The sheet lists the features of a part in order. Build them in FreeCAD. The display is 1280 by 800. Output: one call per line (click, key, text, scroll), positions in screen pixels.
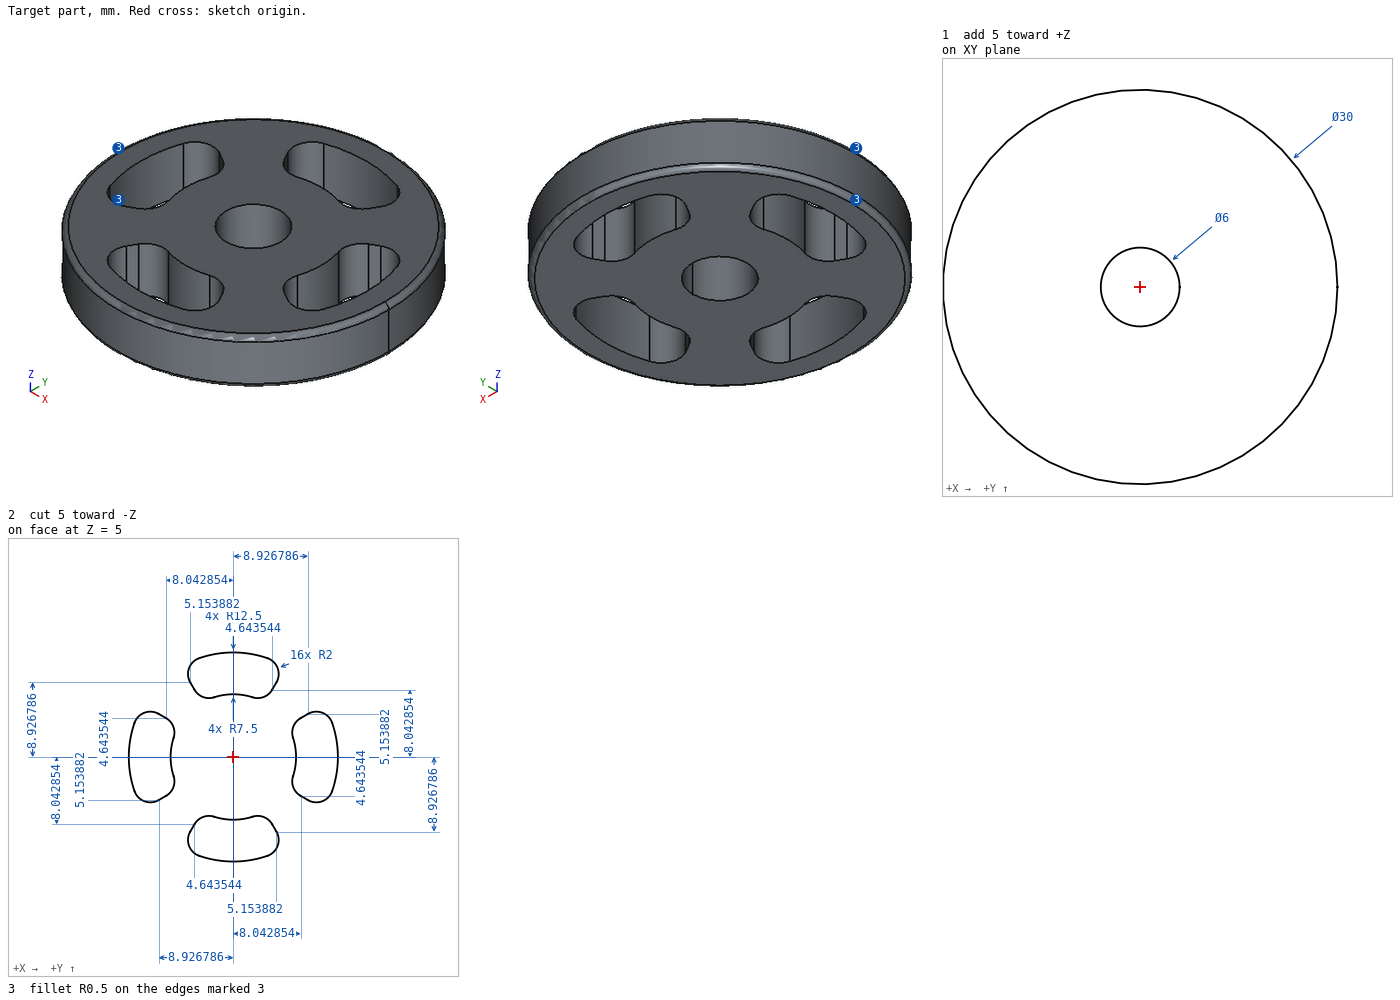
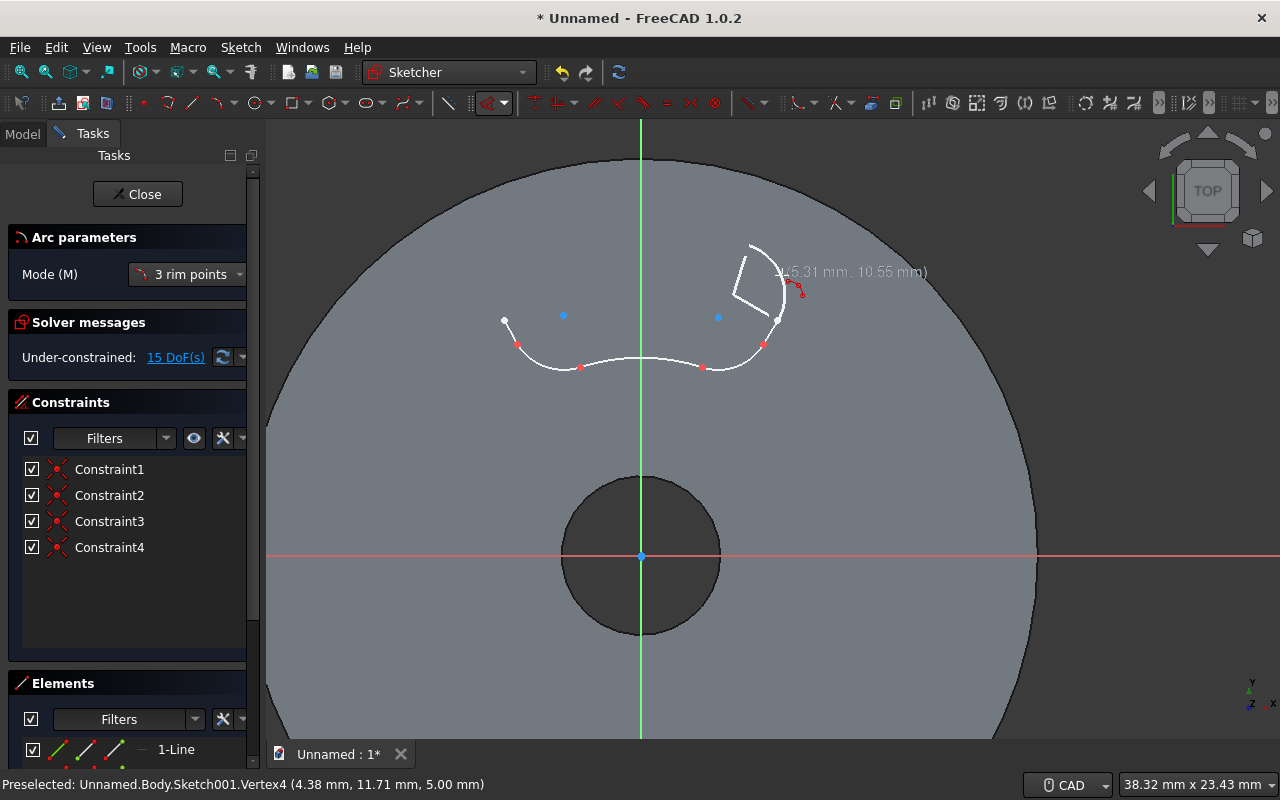
click(781, 274)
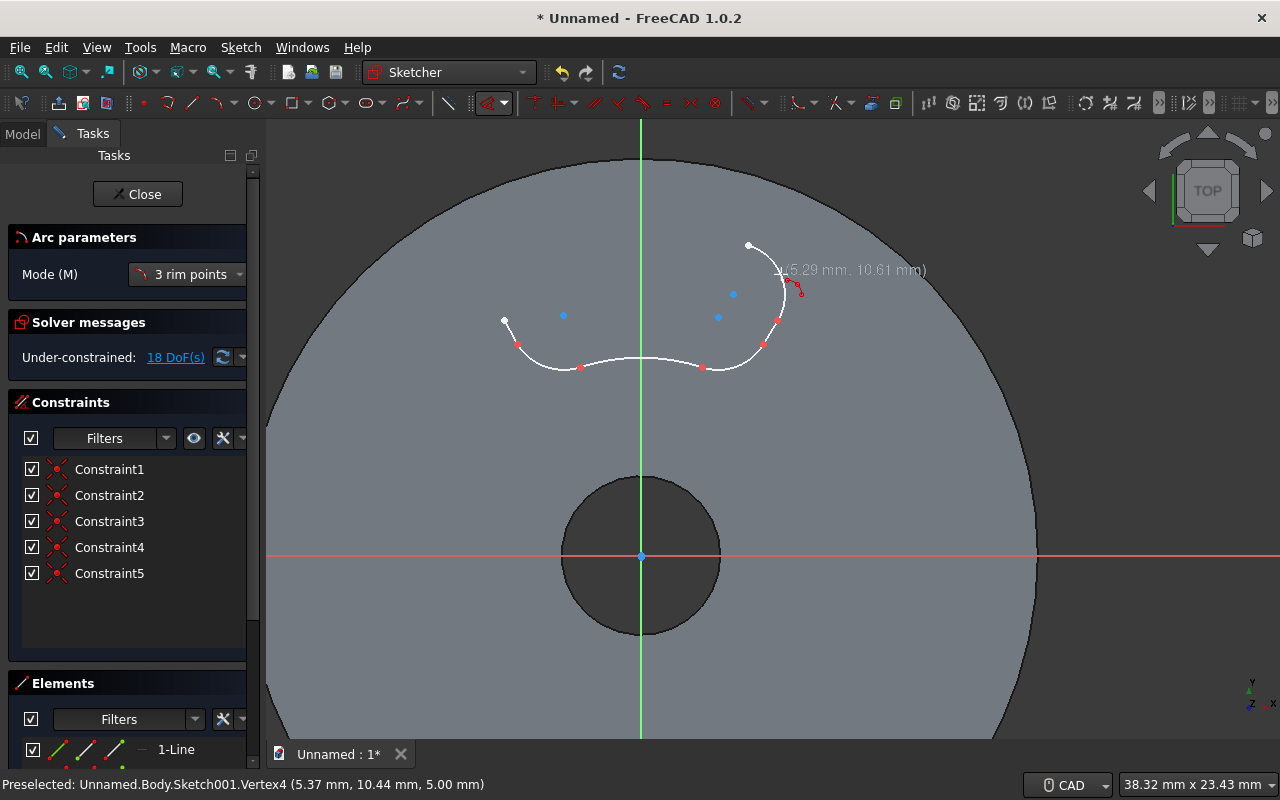
click(749, 246)
click(533, 243)
click(663, 226)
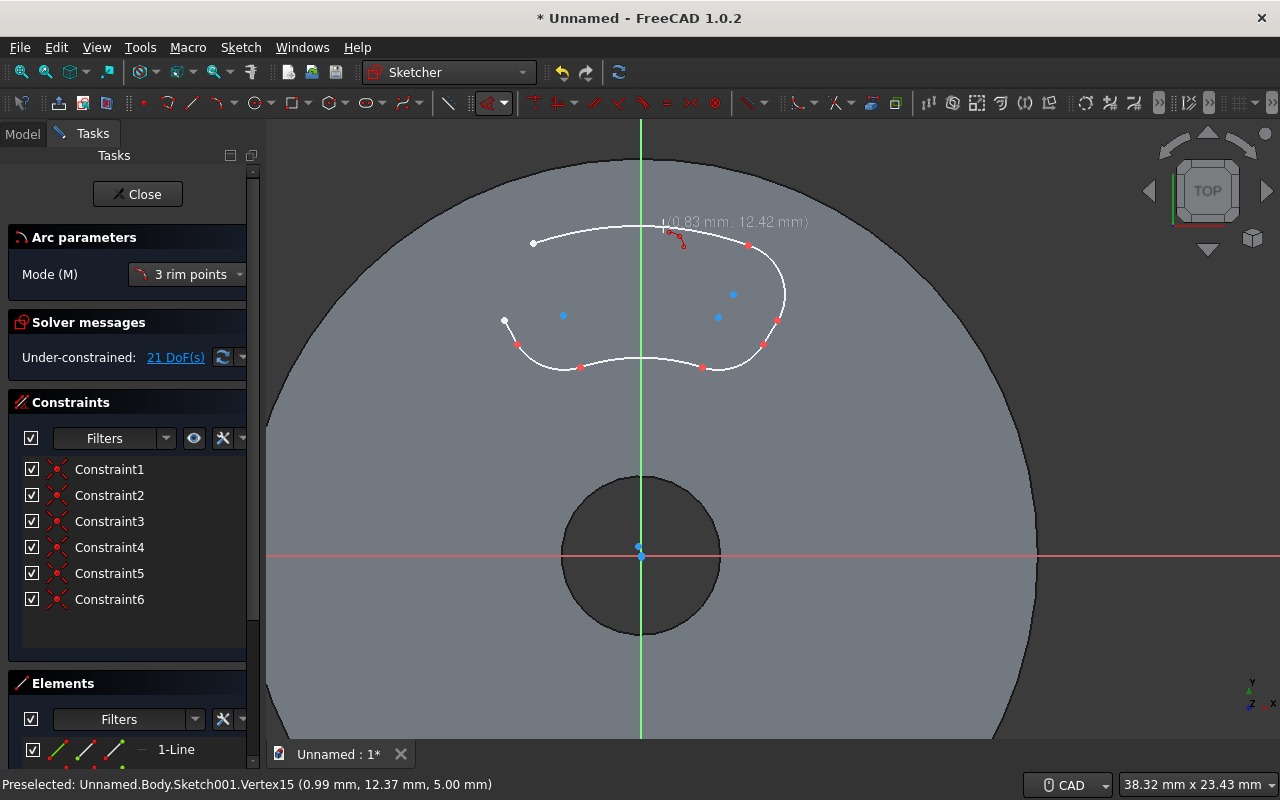
click(533, 244)
click(505, 321)
click(501, 274)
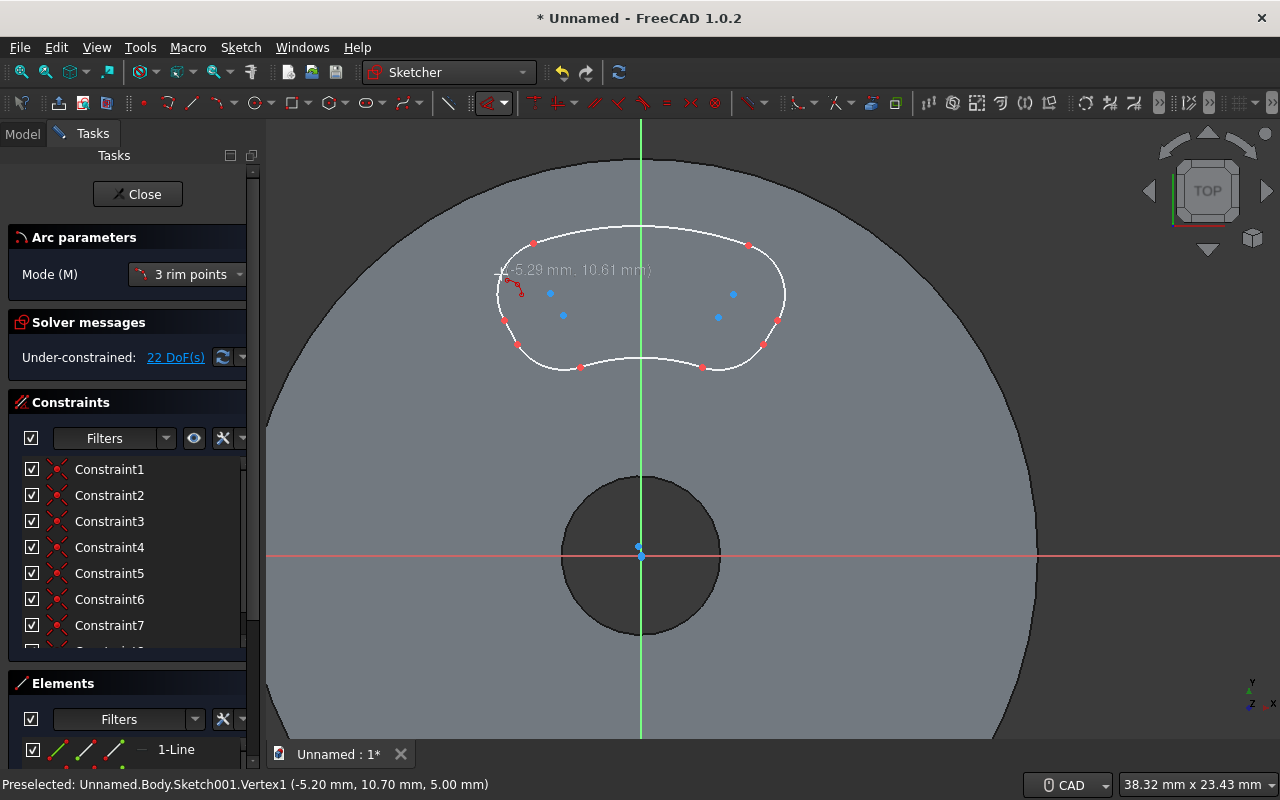
click(192, 104)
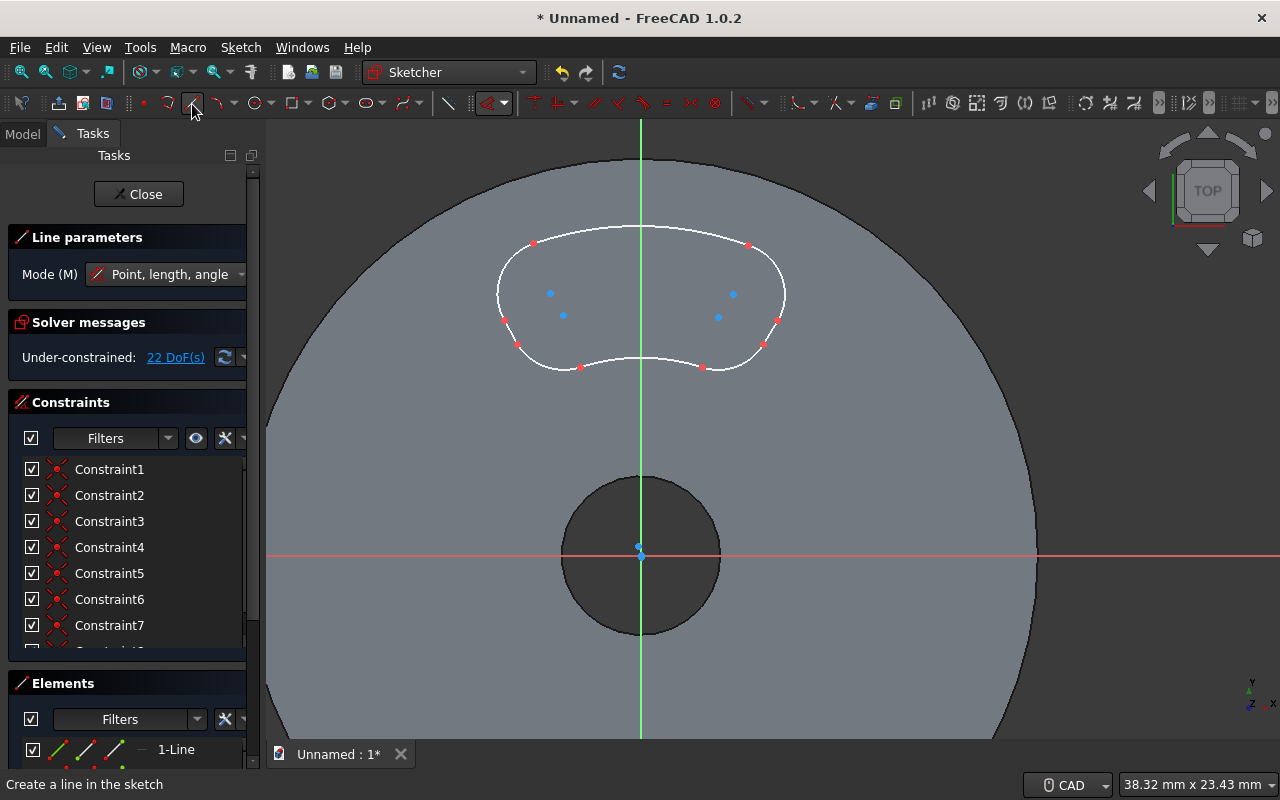
click(877, 419)
click(854, 433)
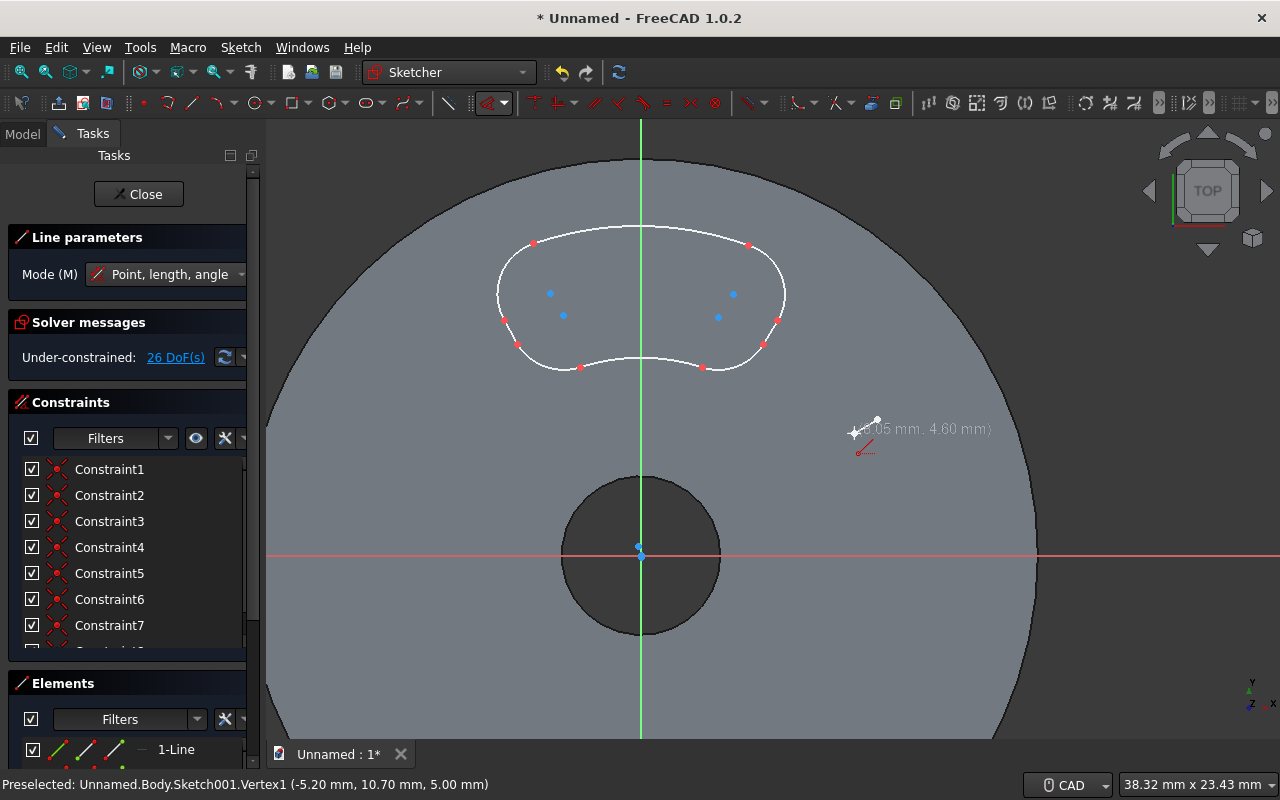
click(854, 678)
click(877, 692)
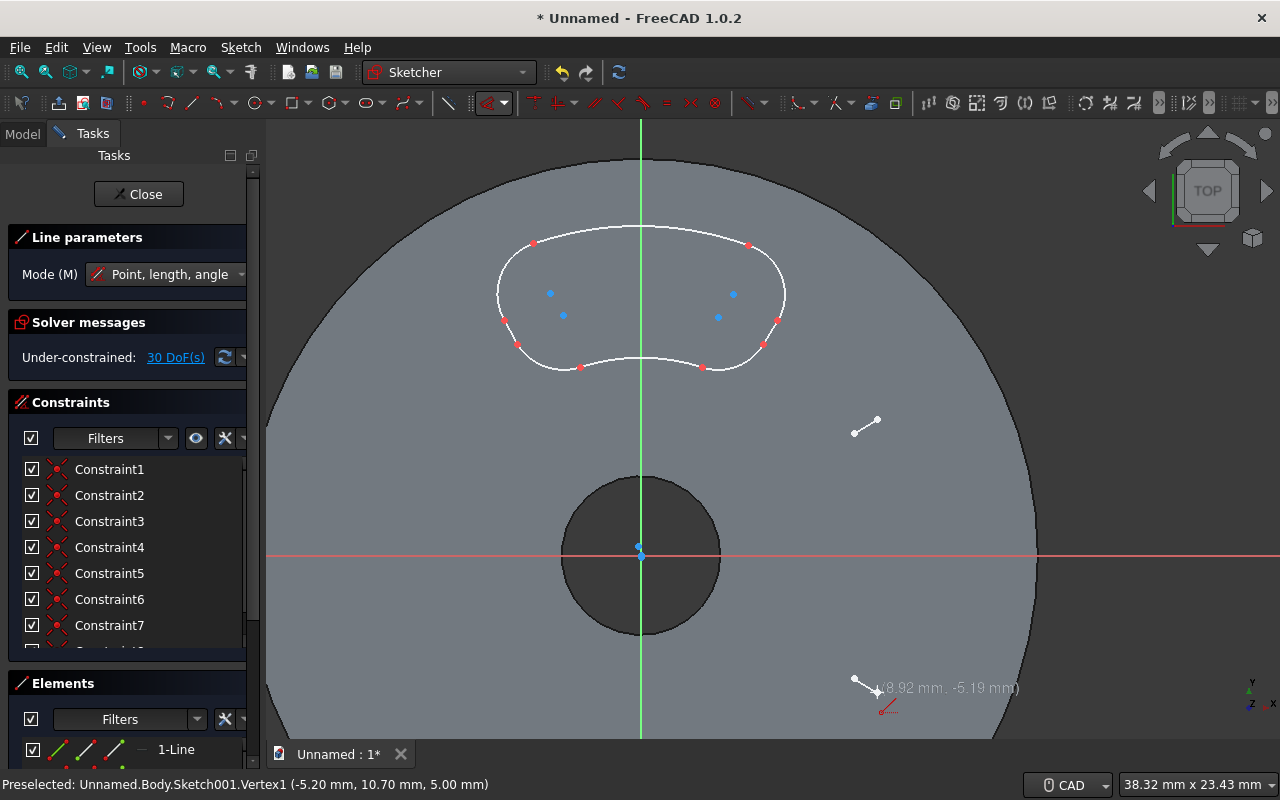
click(218, 104)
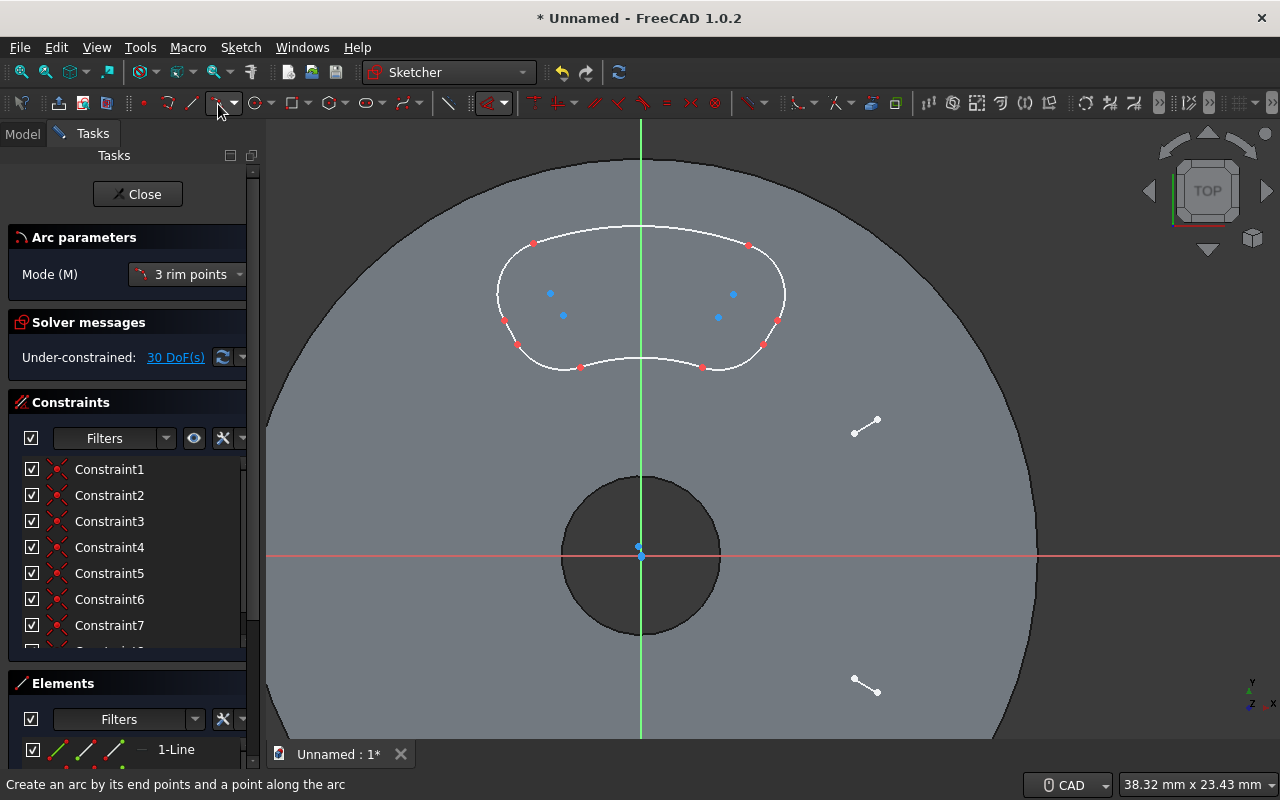
click(854, 434)
click(830, 495)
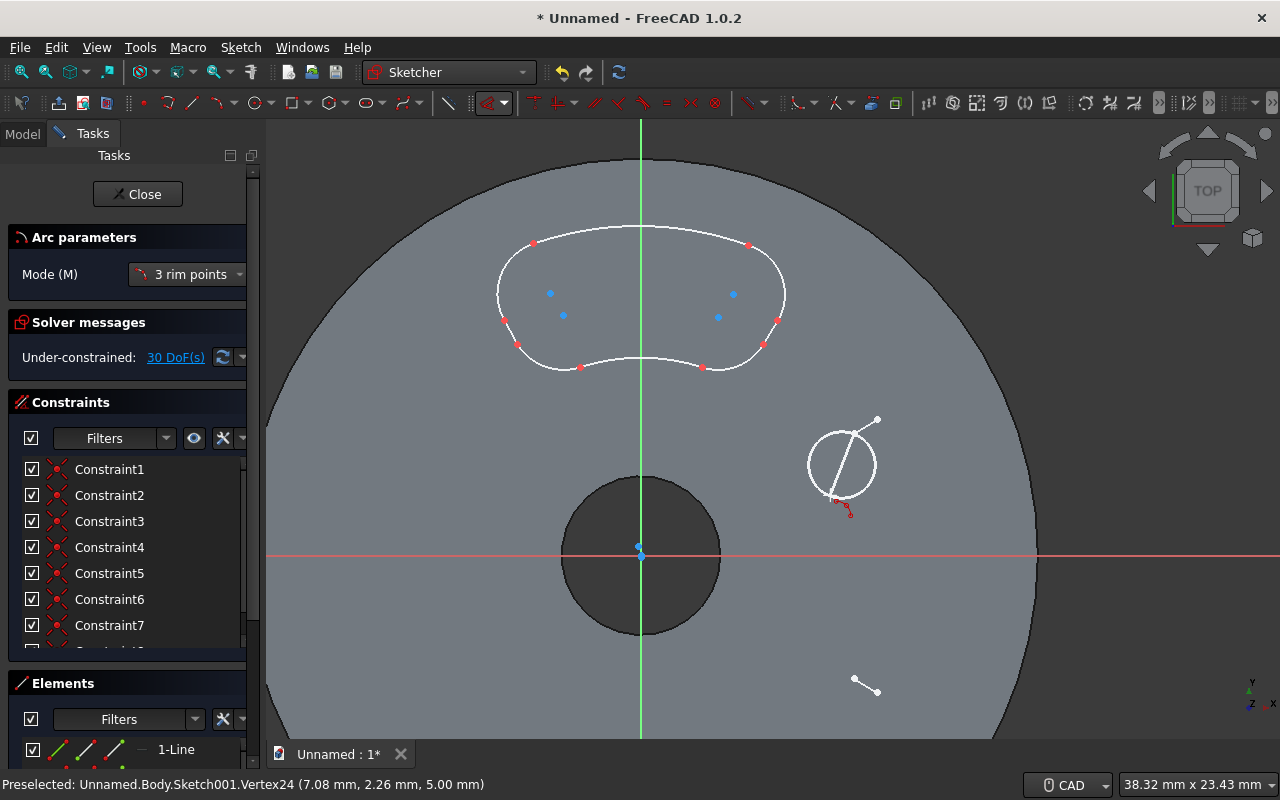
scroll(831, 460, up, 2)